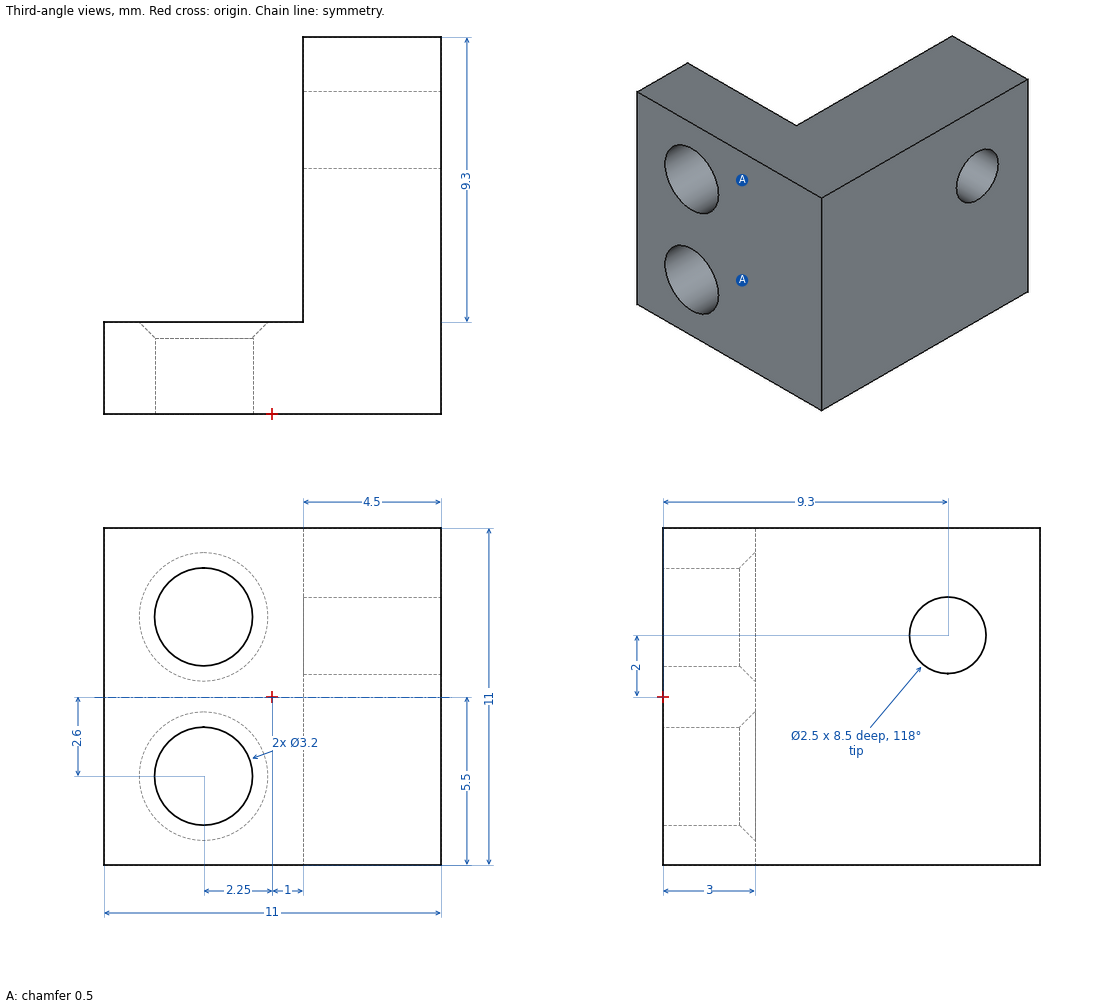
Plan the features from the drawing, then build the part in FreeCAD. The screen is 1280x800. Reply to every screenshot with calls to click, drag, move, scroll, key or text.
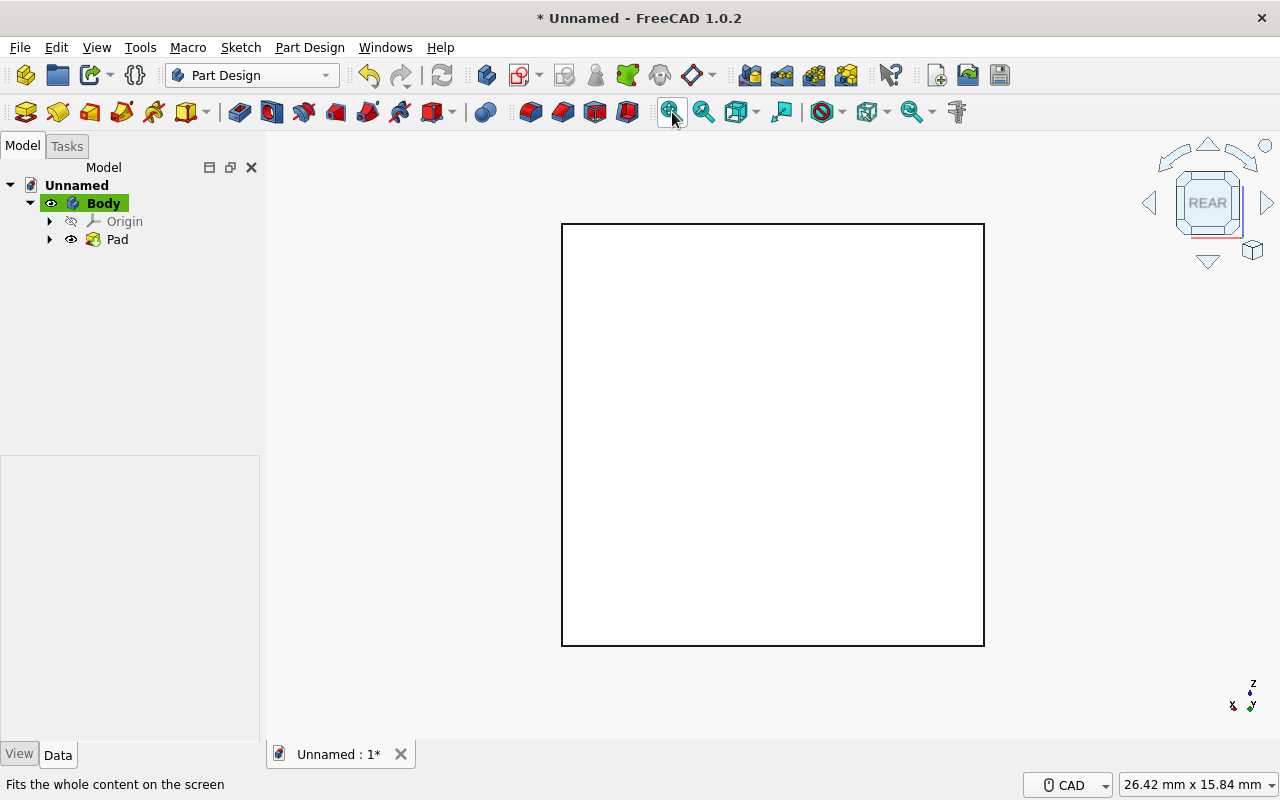
click(773, 434)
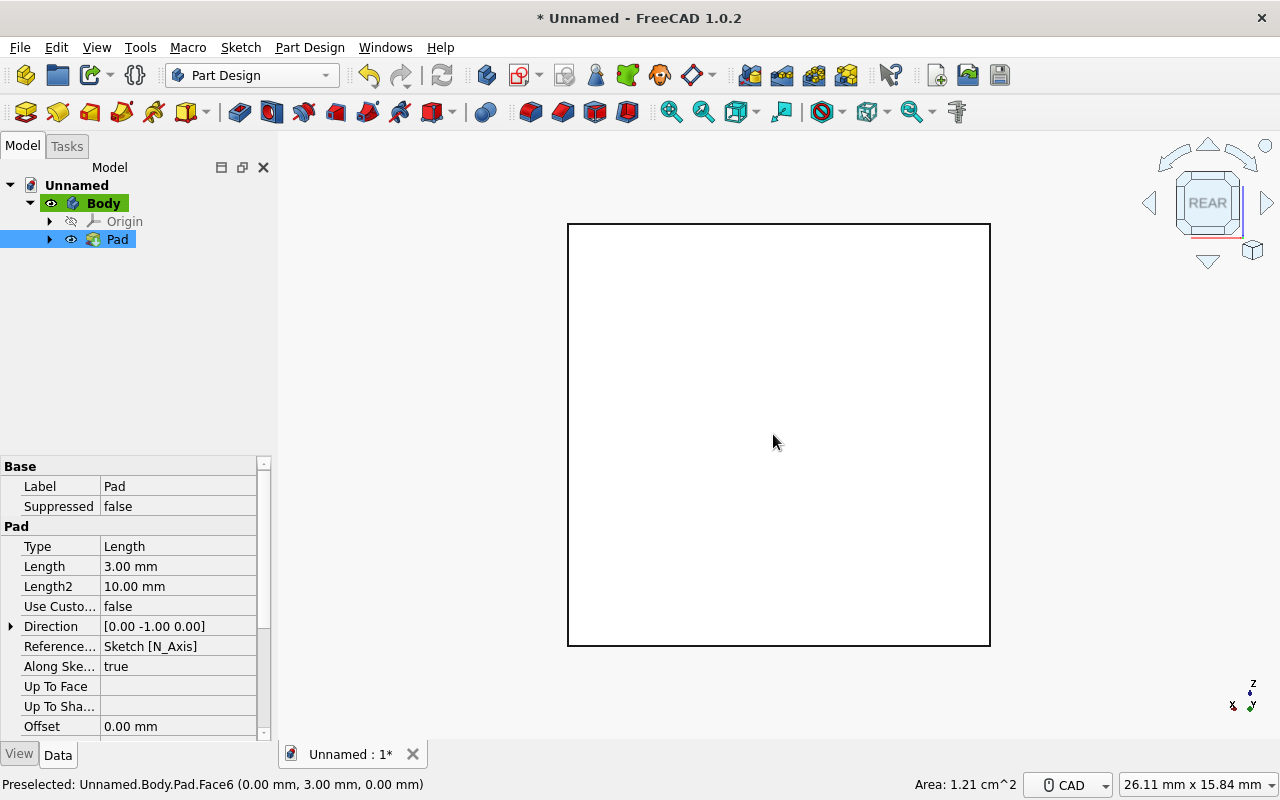
click(520, 76)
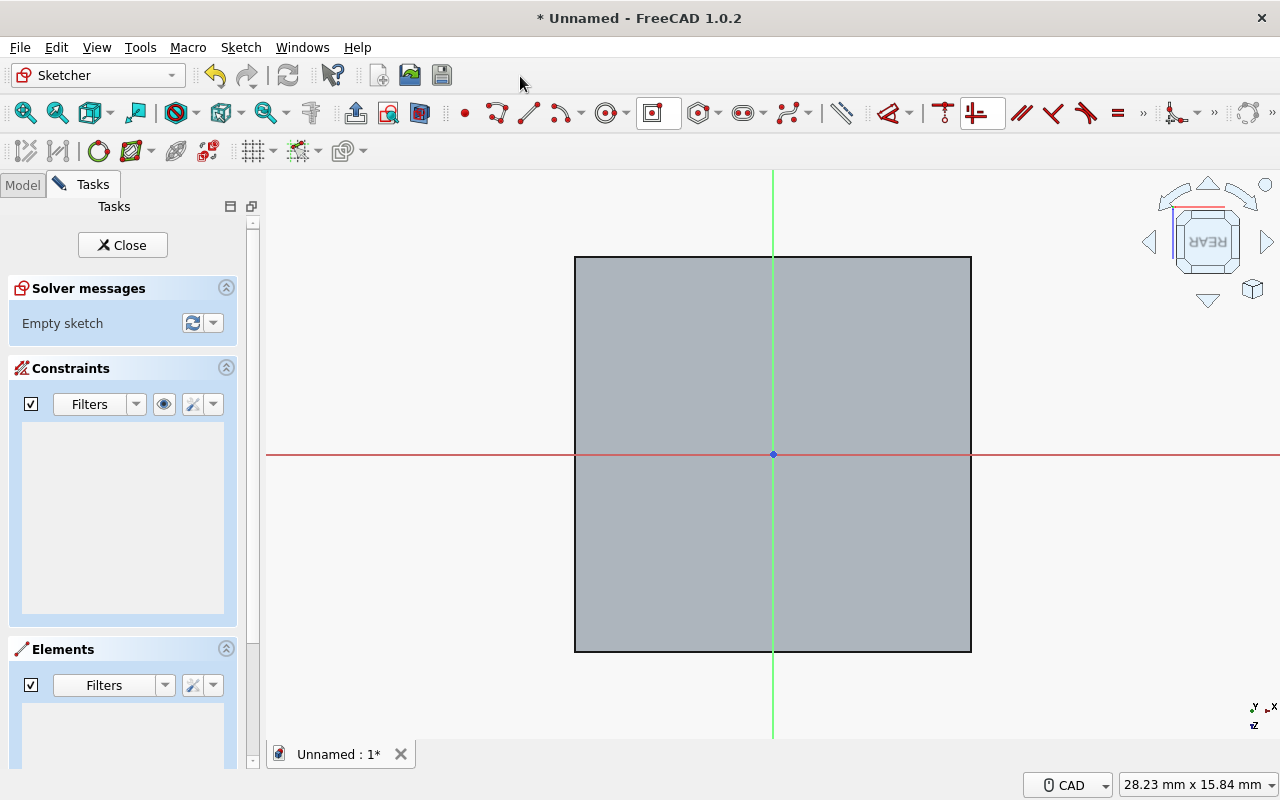
click(676, 114)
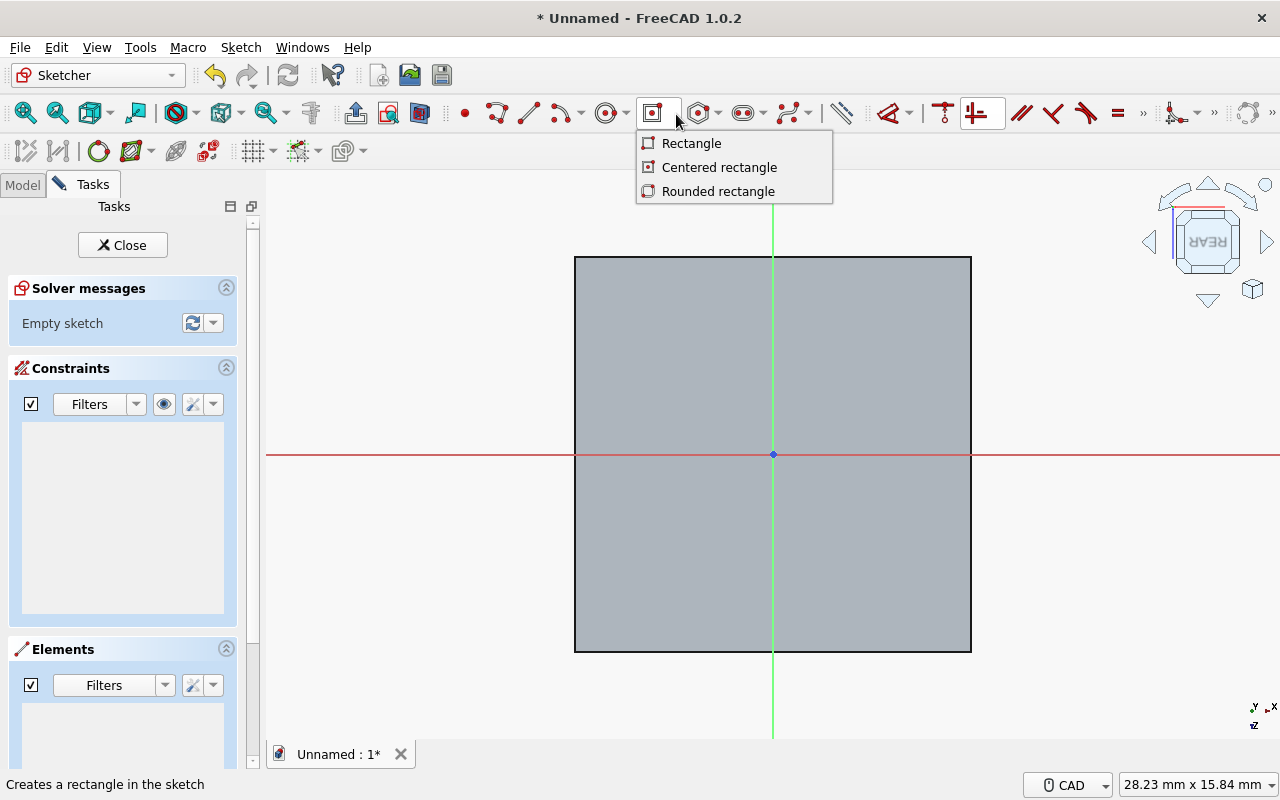
click(734, 143)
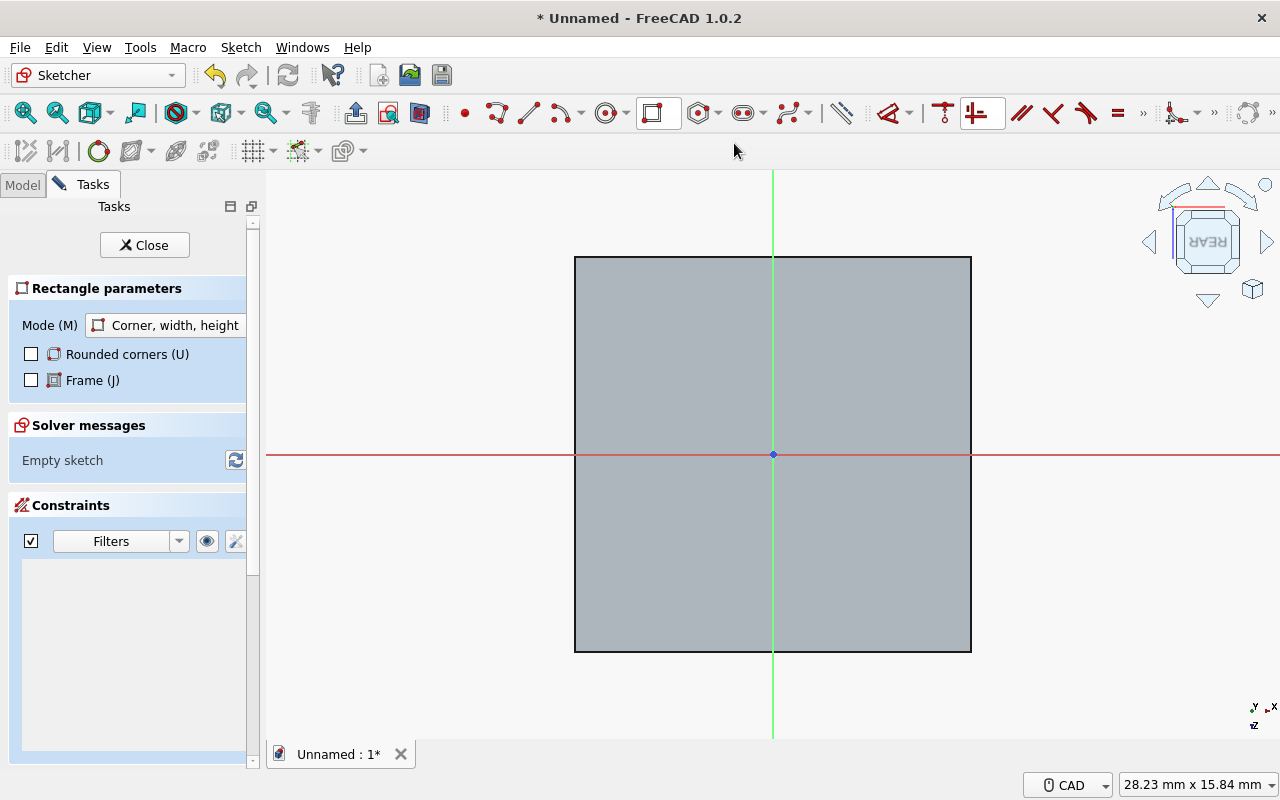
click(809, 257)
click(971, 652)
key(Escape)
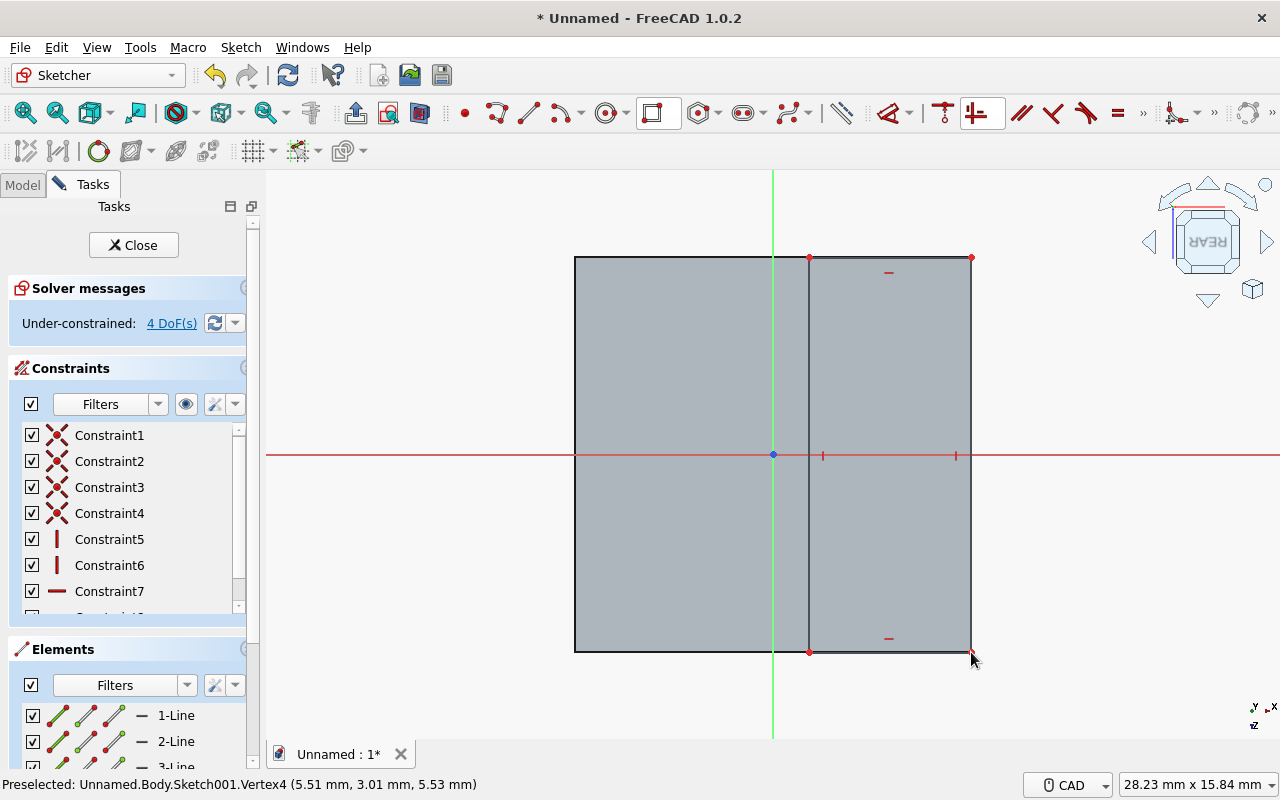
click(888, 114)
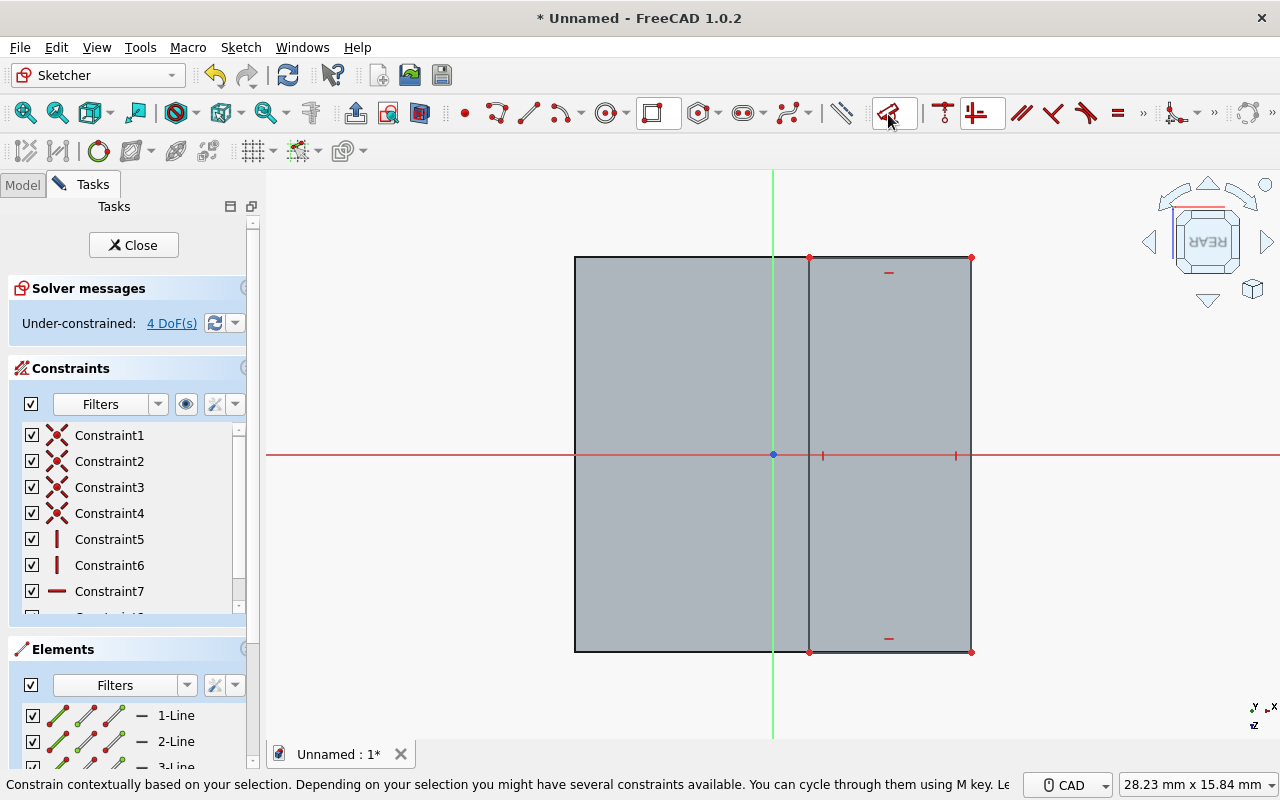
click(809, 376)
click(843, 365)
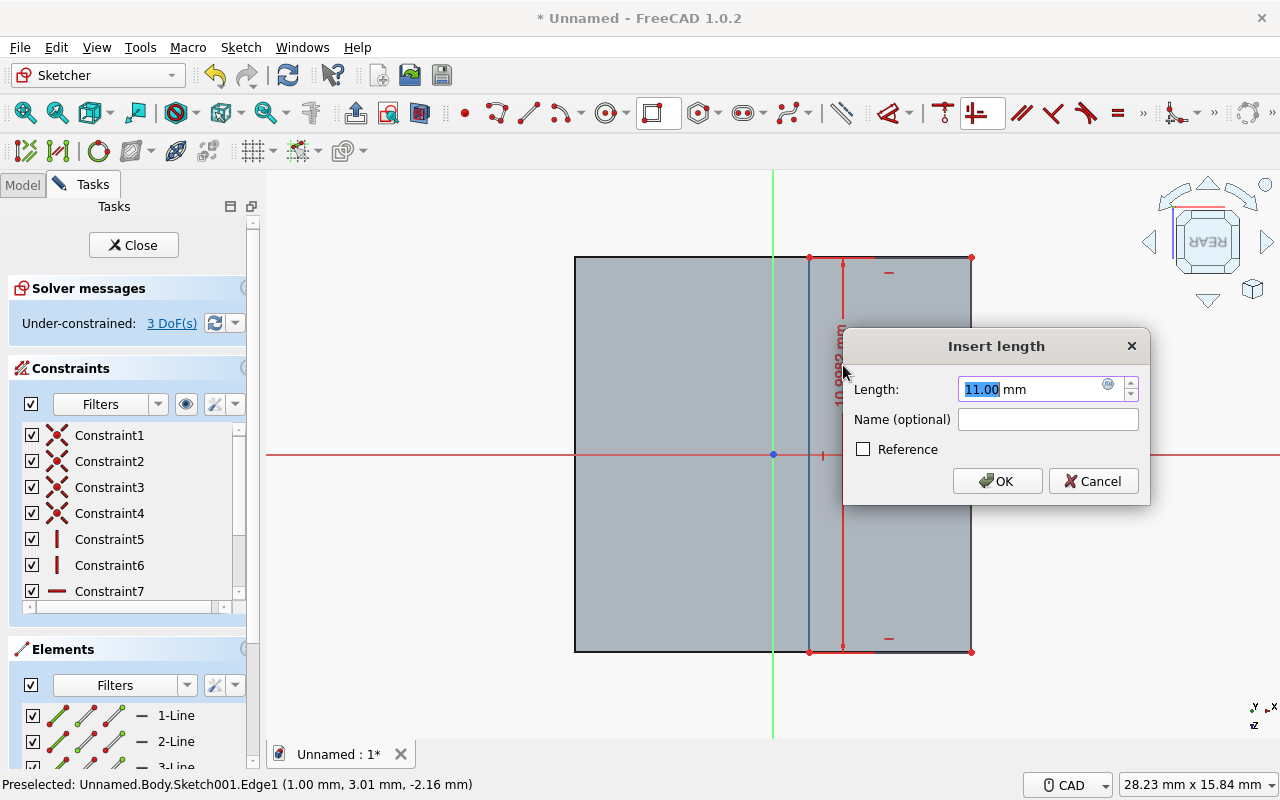
text(11)
key(Return)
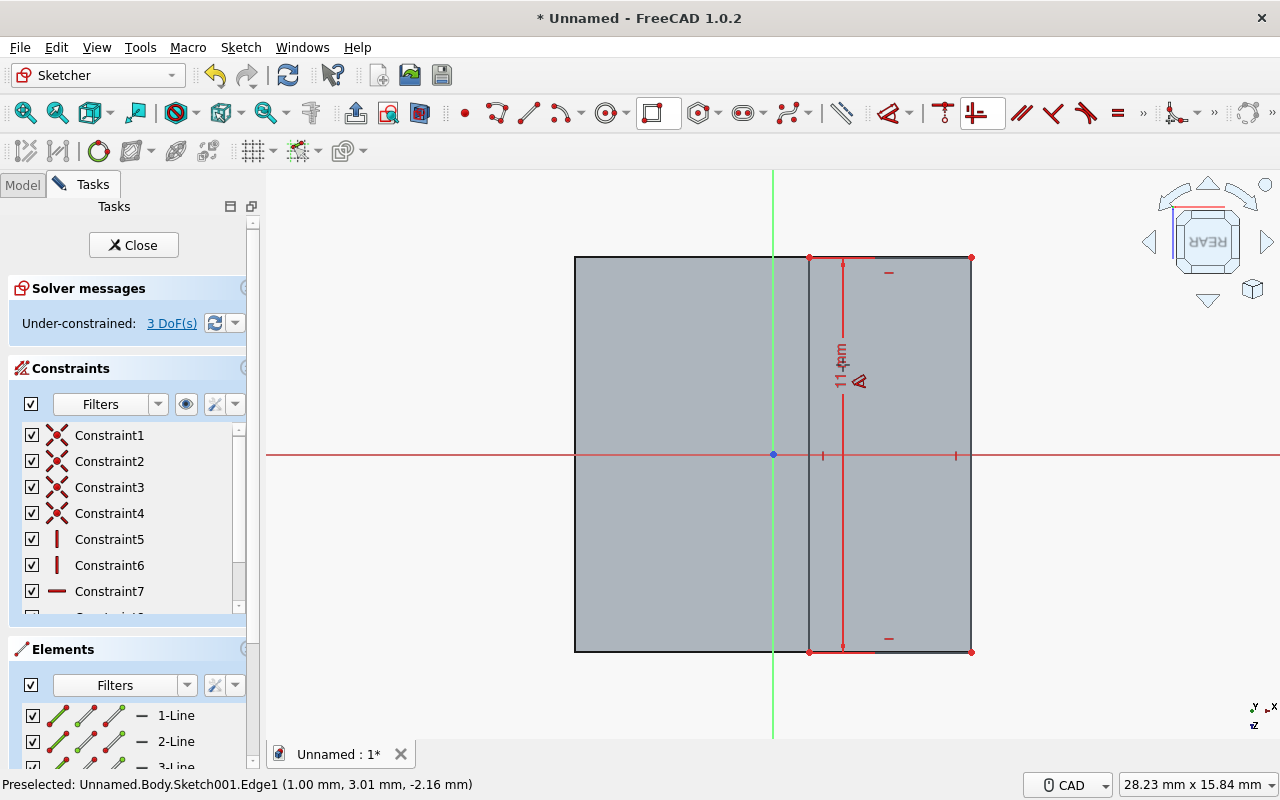
click(809, 258)
click(791, 224)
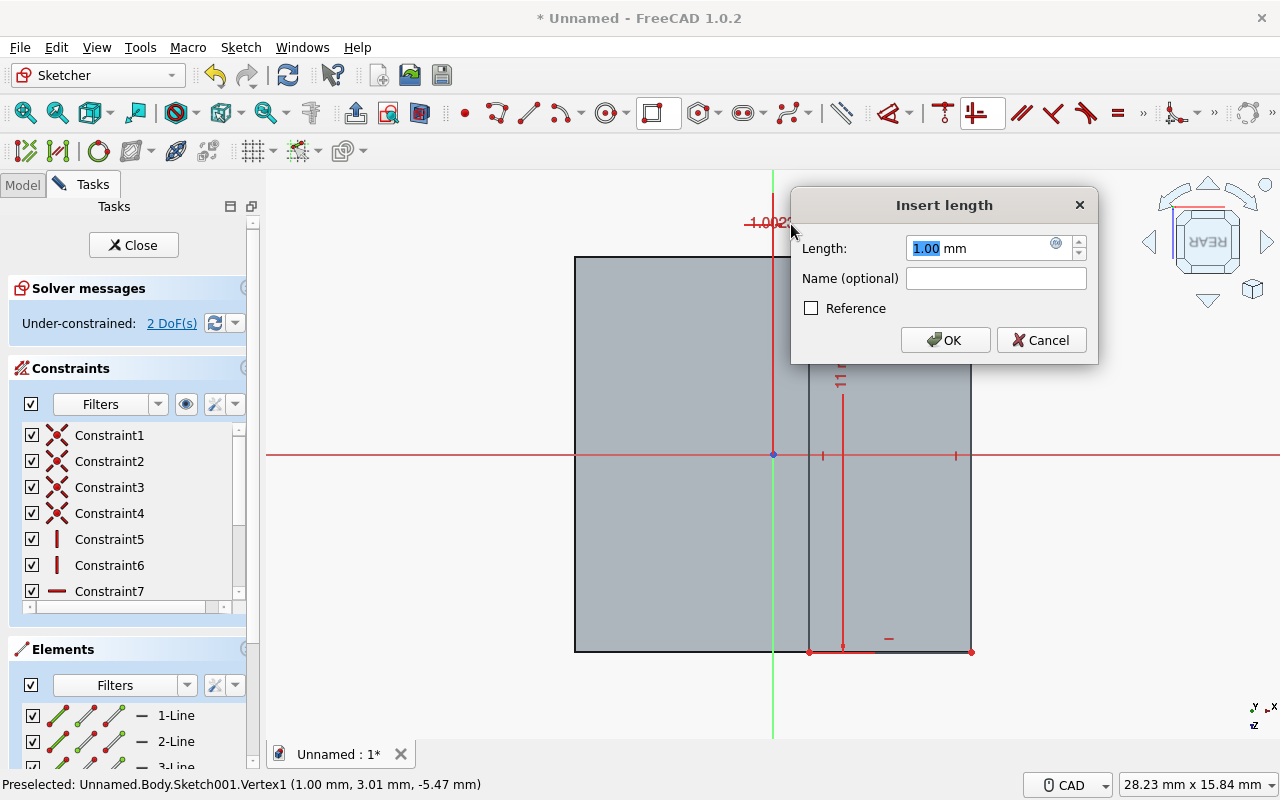
text(1)
key(Return)